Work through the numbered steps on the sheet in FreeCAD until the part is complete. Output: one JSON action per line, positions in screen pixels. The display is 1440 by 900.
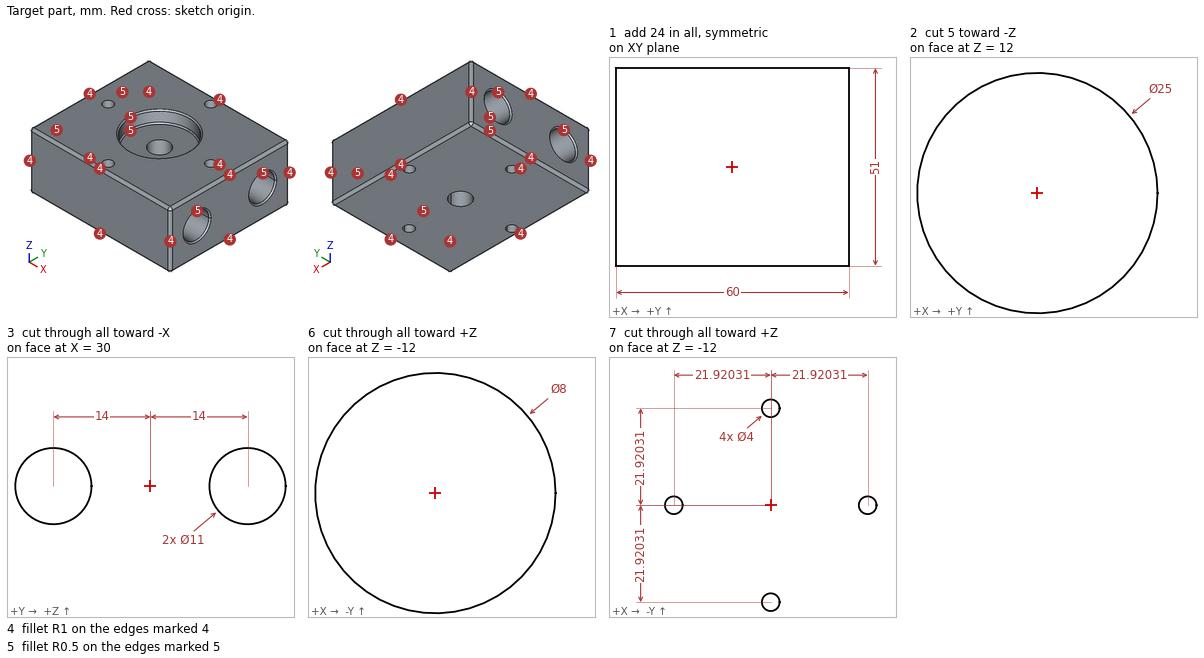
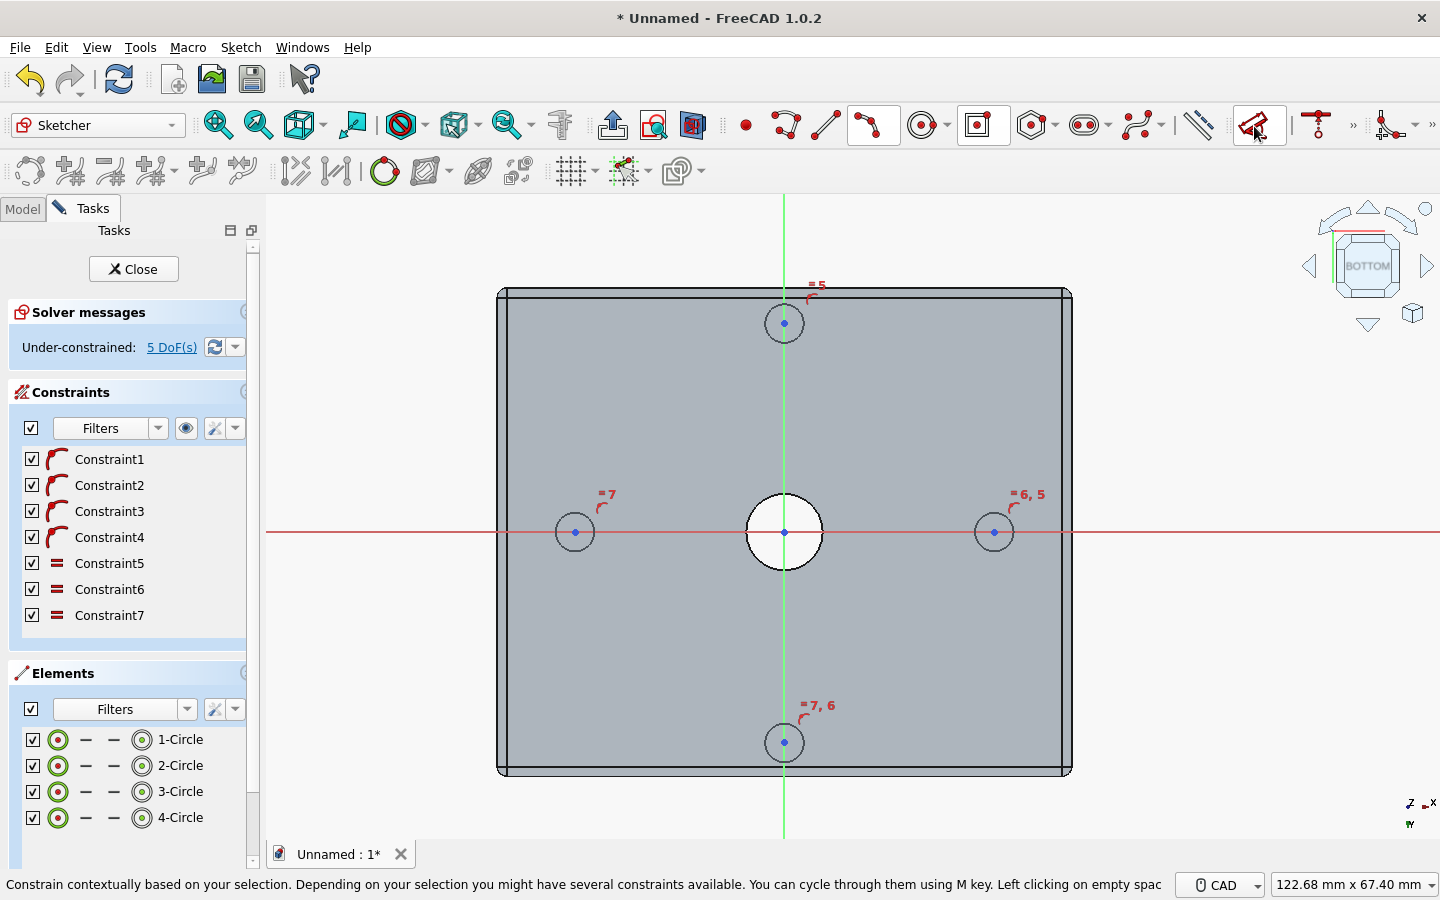
{"action": "left_click", "coordinate": [798, 310]}
{"action": "left_click", "coordinate": [821, 287]}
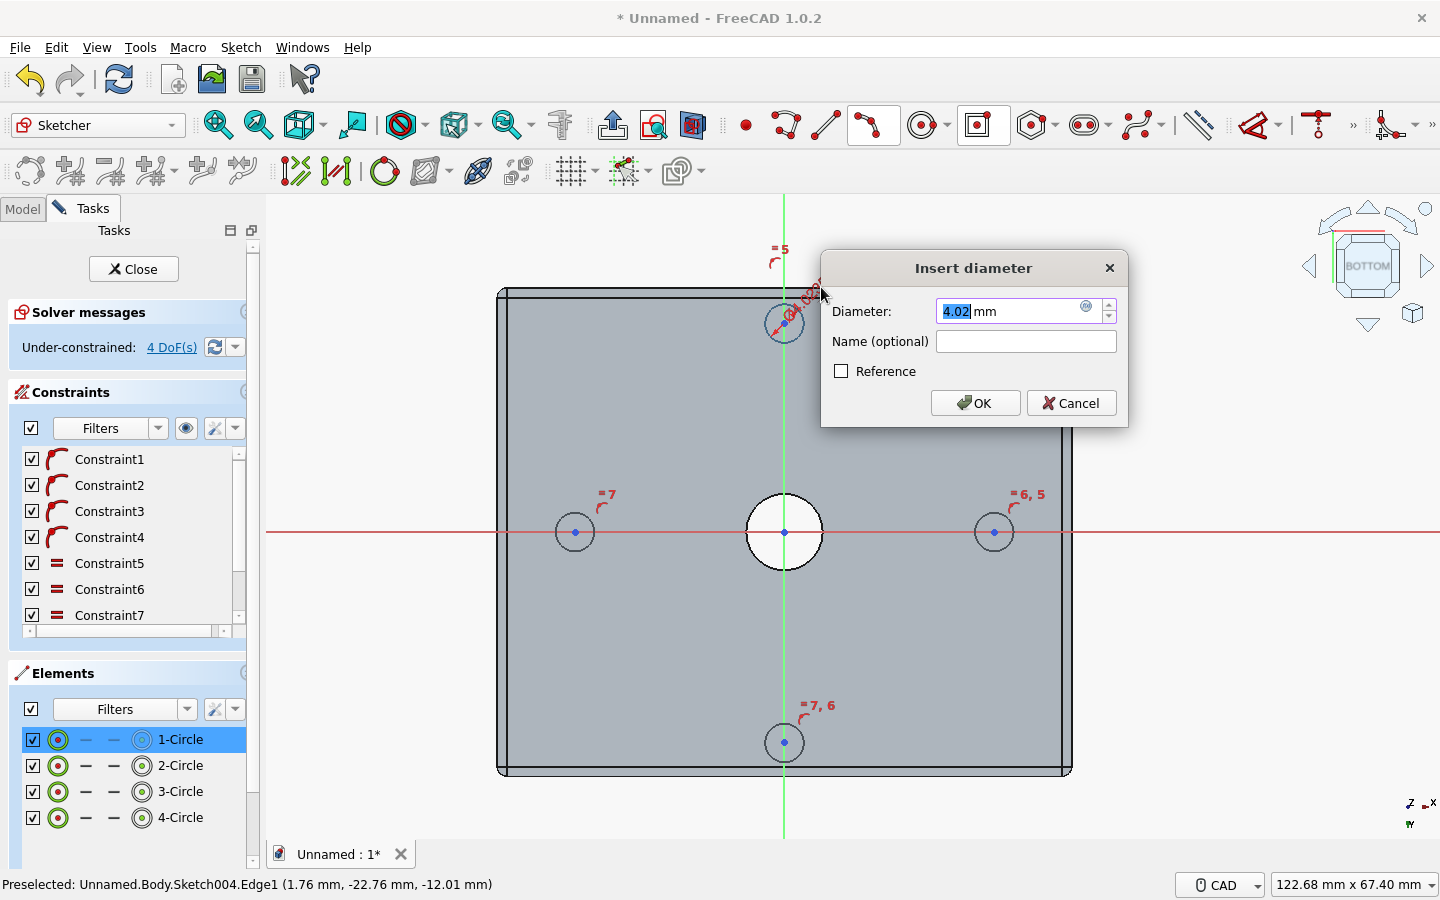
{"action": "type", "text": "4"}
{"action": "key", "text": "Return"}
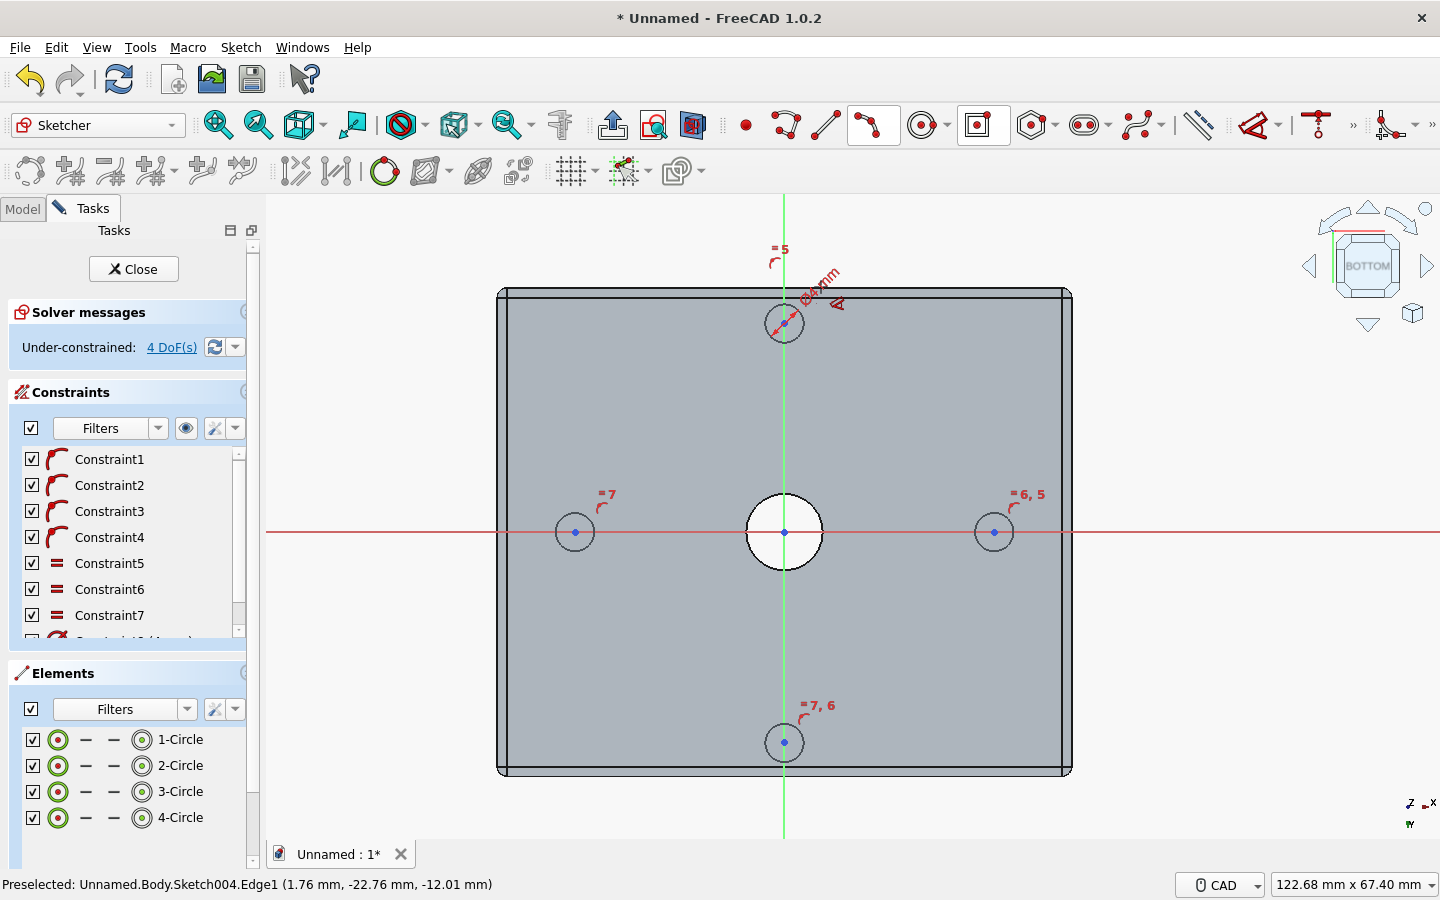
{"action": "left_click", "coordinate": [784, 324]}
{"action": "left_click", "coordinate": [818, 428]}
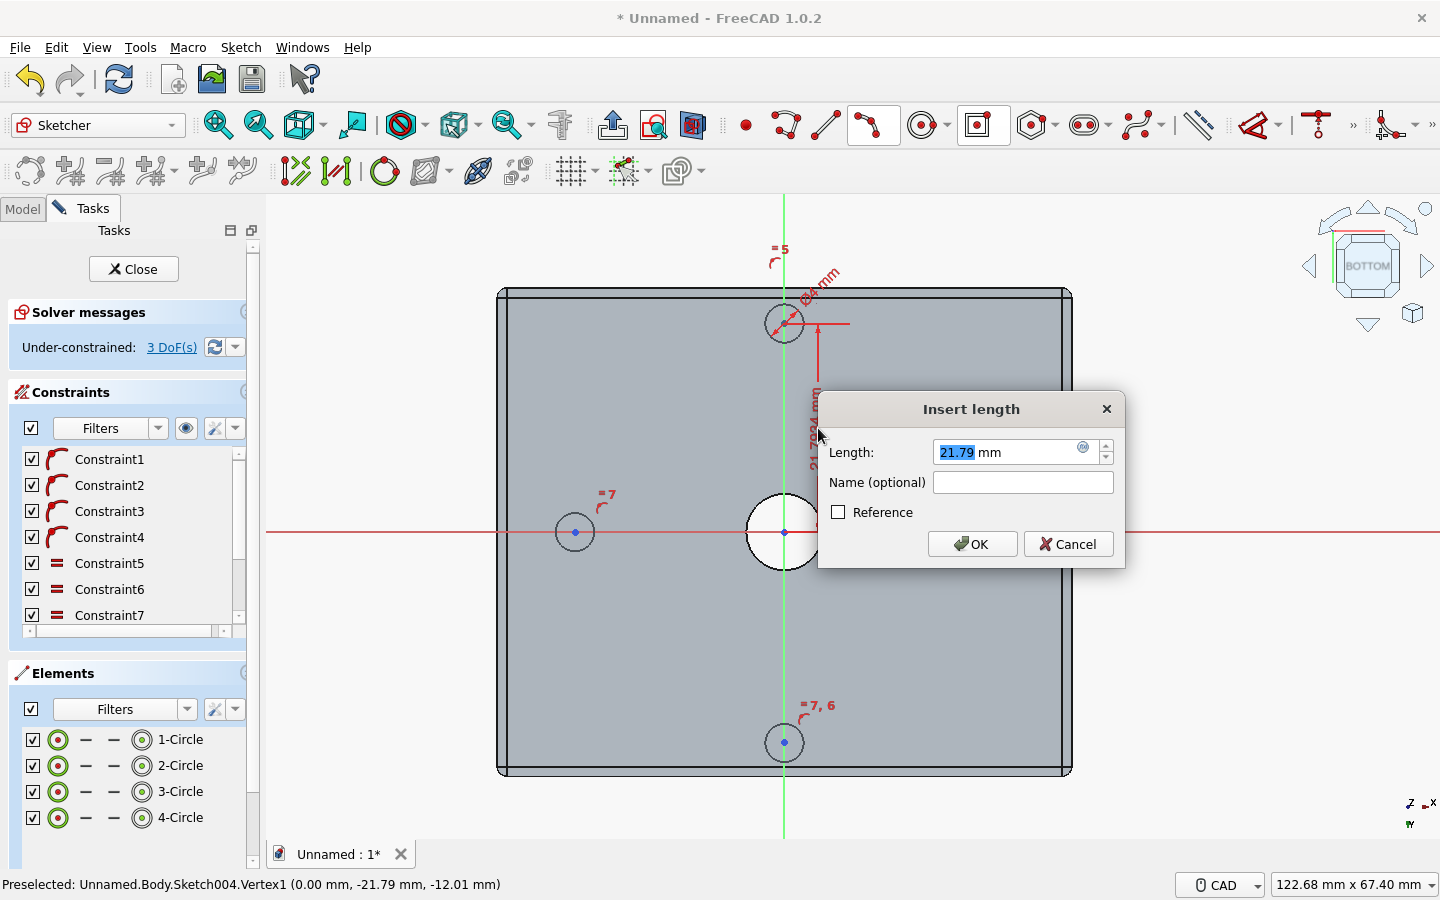
{"action": "type", "text": "21.92031"}
{"action": "key", "text": "Return"}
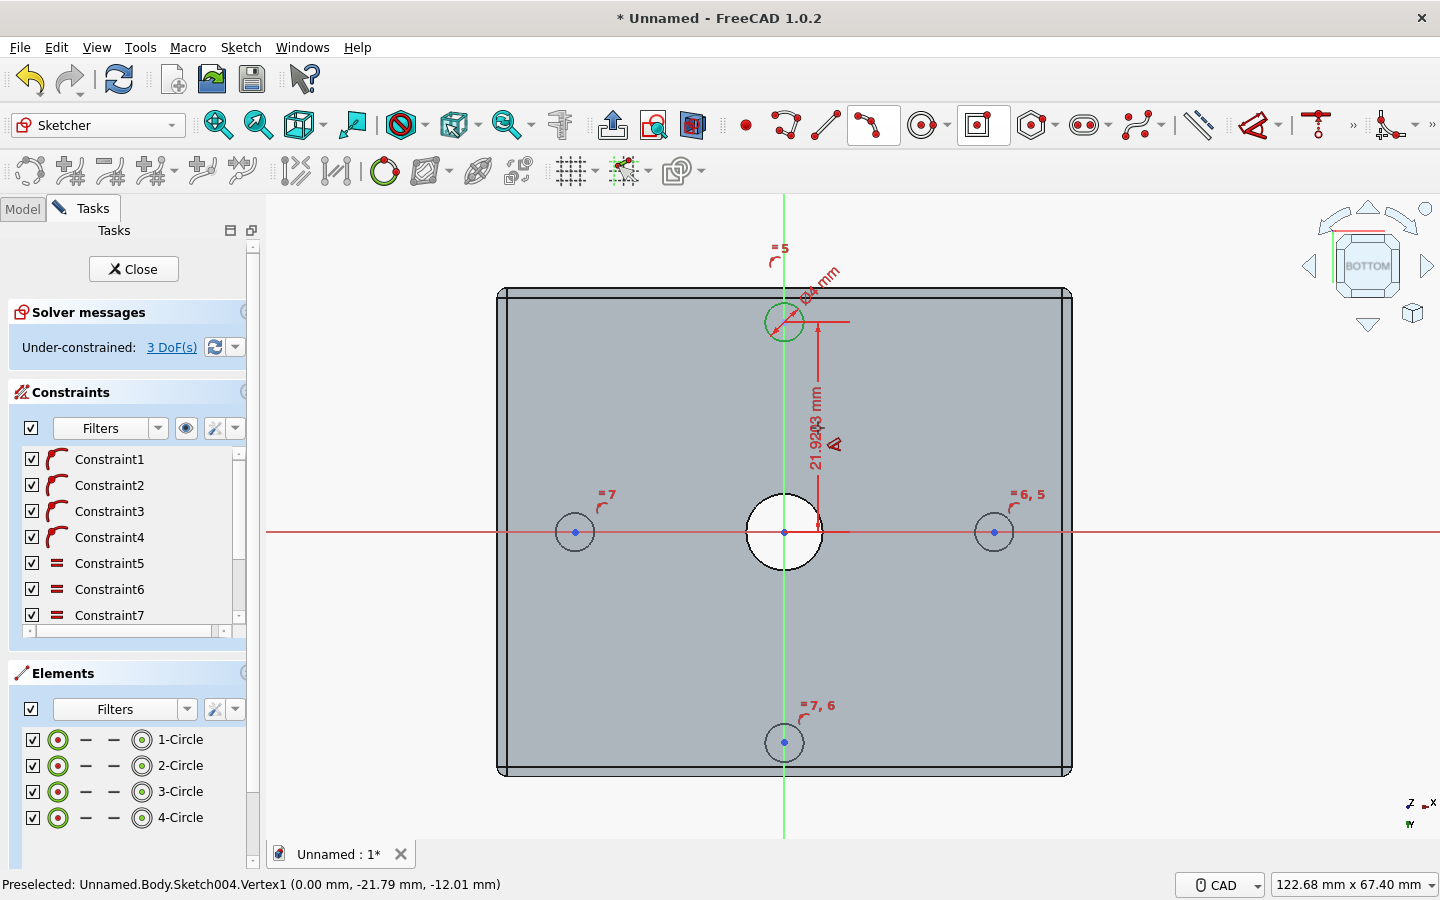
{"action": "left_click", "coordinate": [994, 532]}
{"action": "left_click", "coordinate": [889, 566]}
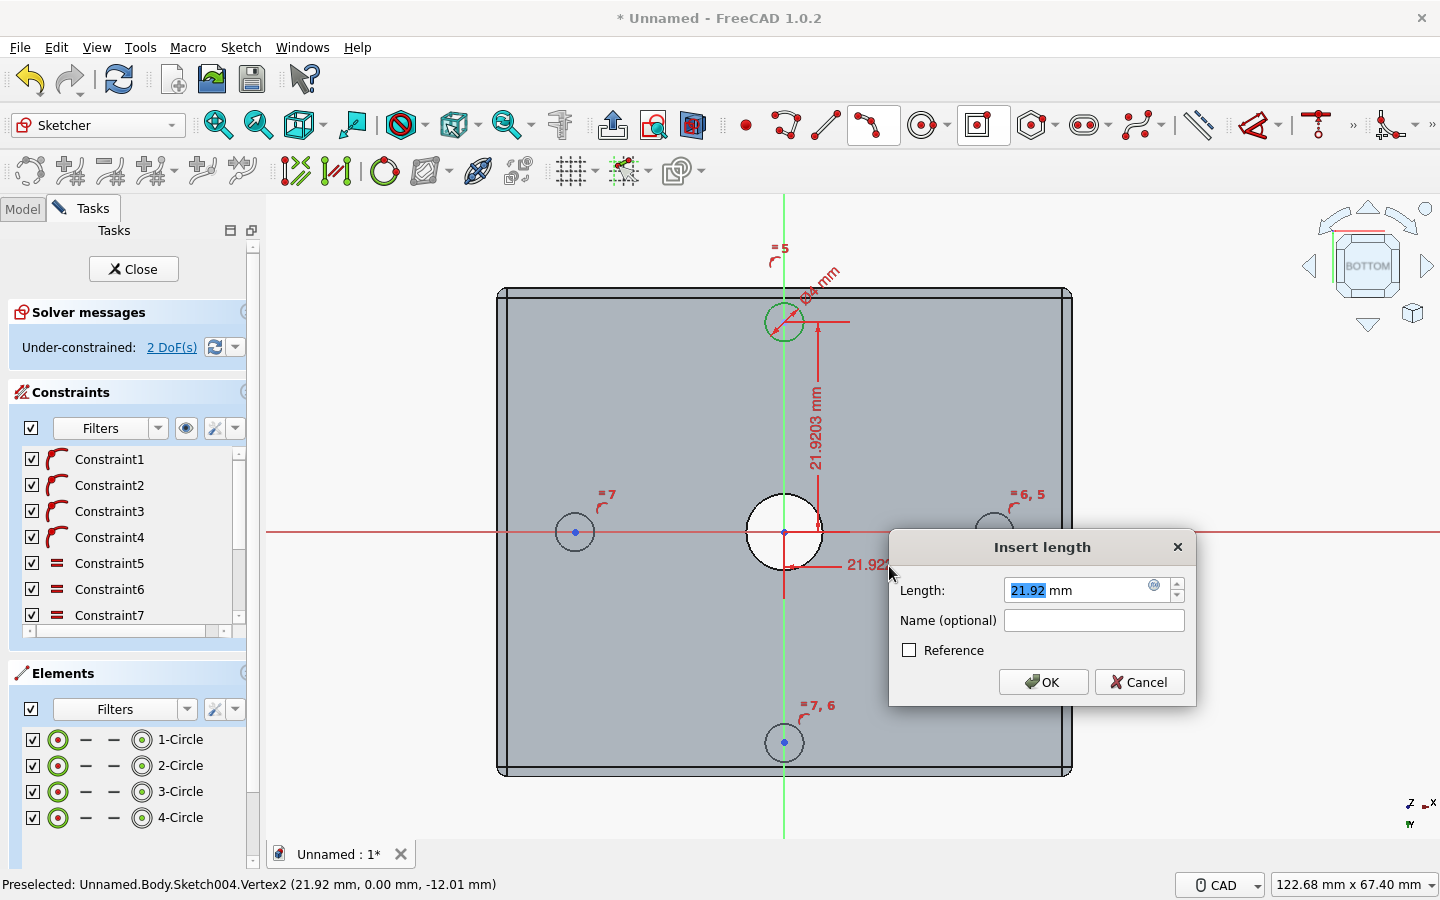
{"action": "type", "text": "21.92031"}
{"action": "key", "text": "Return"}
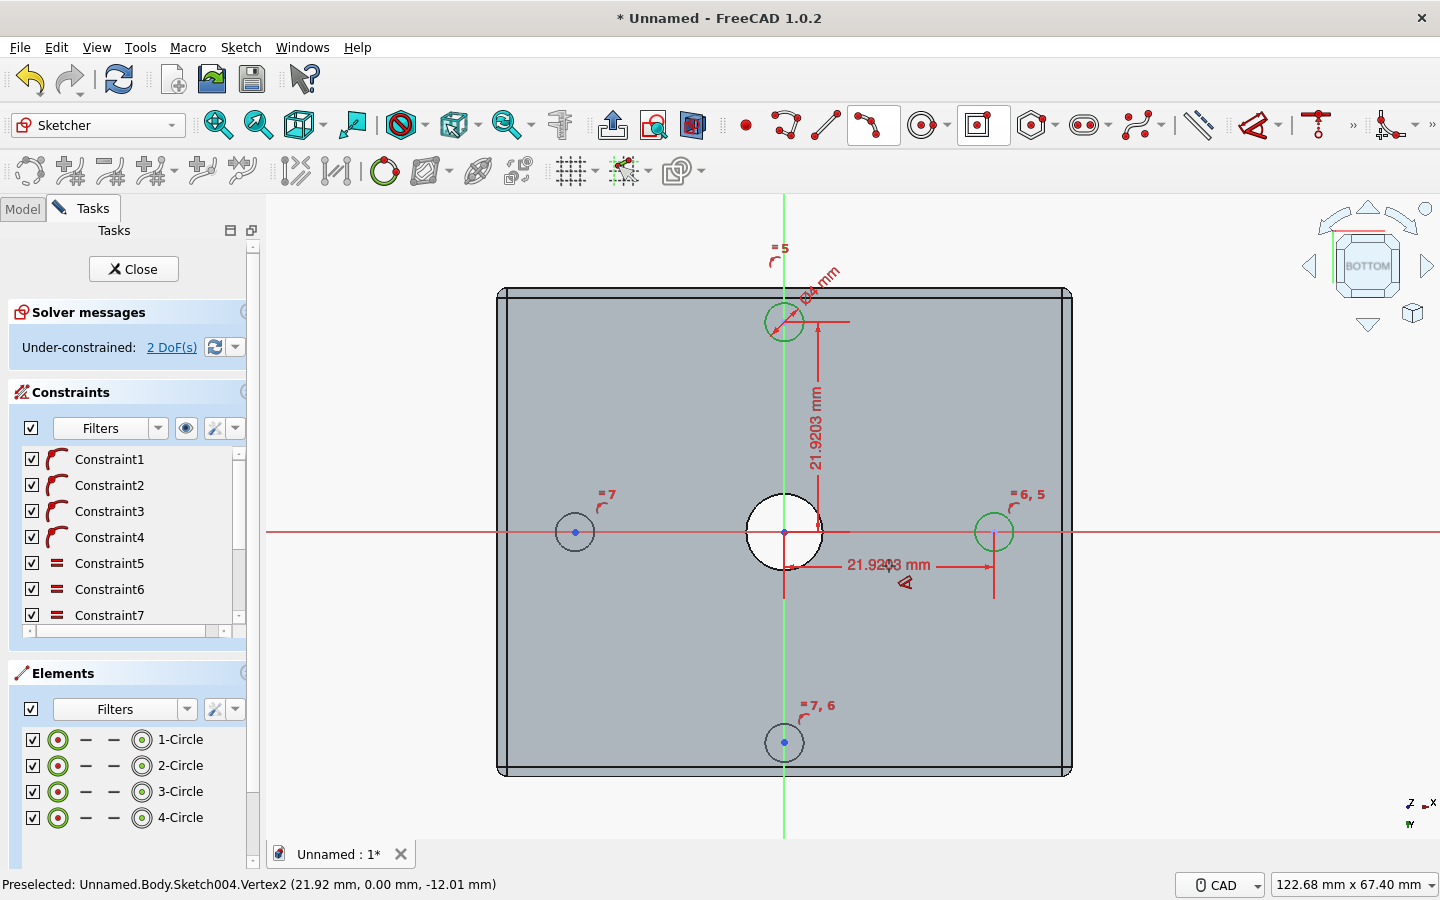
{"action": "left_click", "coordinate": [784, 743]}
{"action": "left_click", "coordinate": [818, 638]}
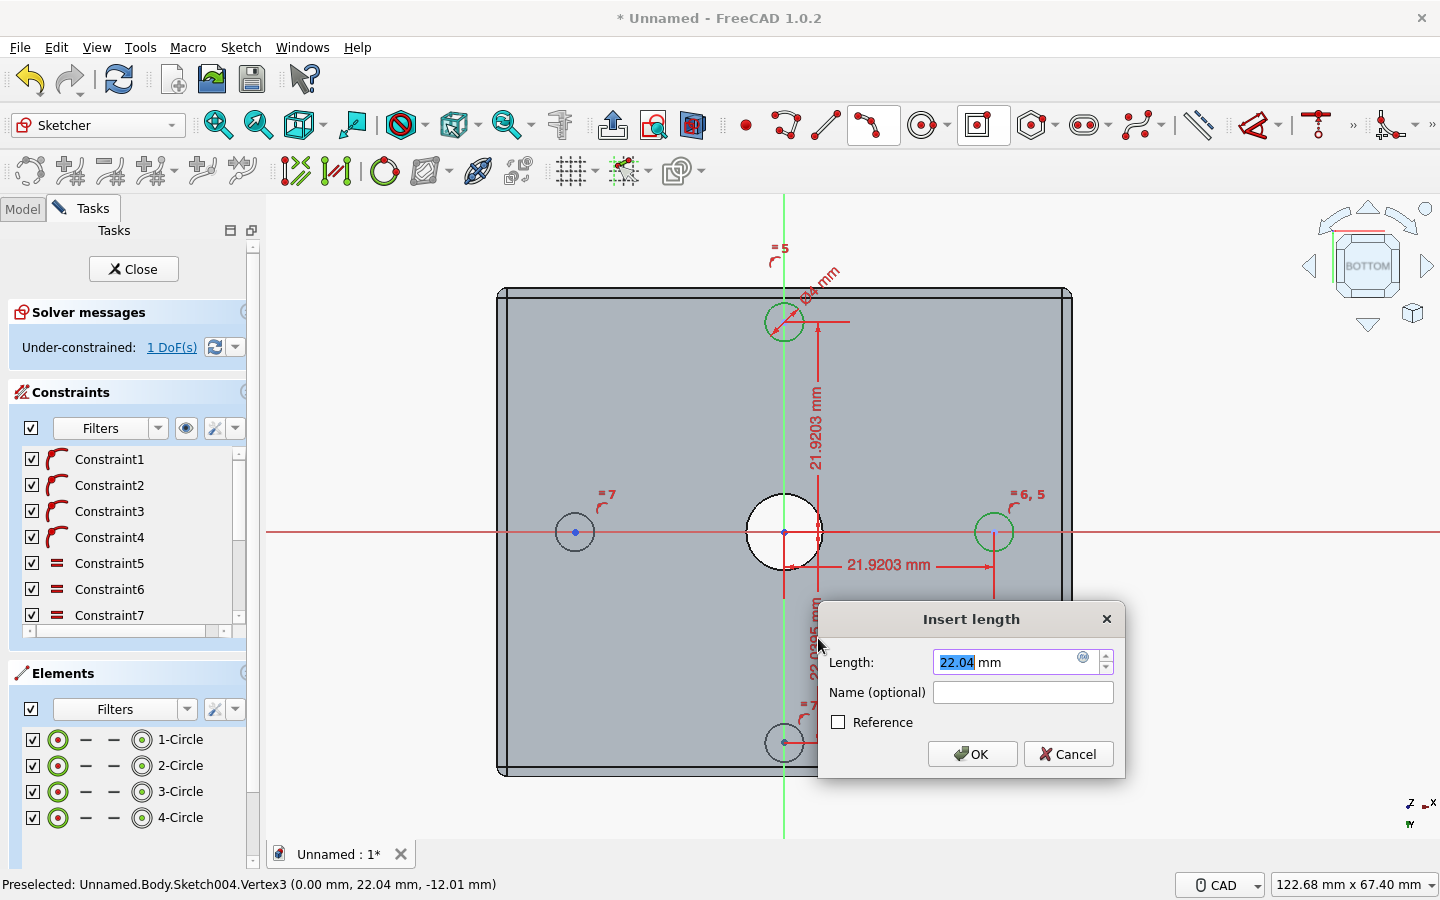
{"action": "type", "text": "21.92031"}
{"action": "key", "text": "Return"}